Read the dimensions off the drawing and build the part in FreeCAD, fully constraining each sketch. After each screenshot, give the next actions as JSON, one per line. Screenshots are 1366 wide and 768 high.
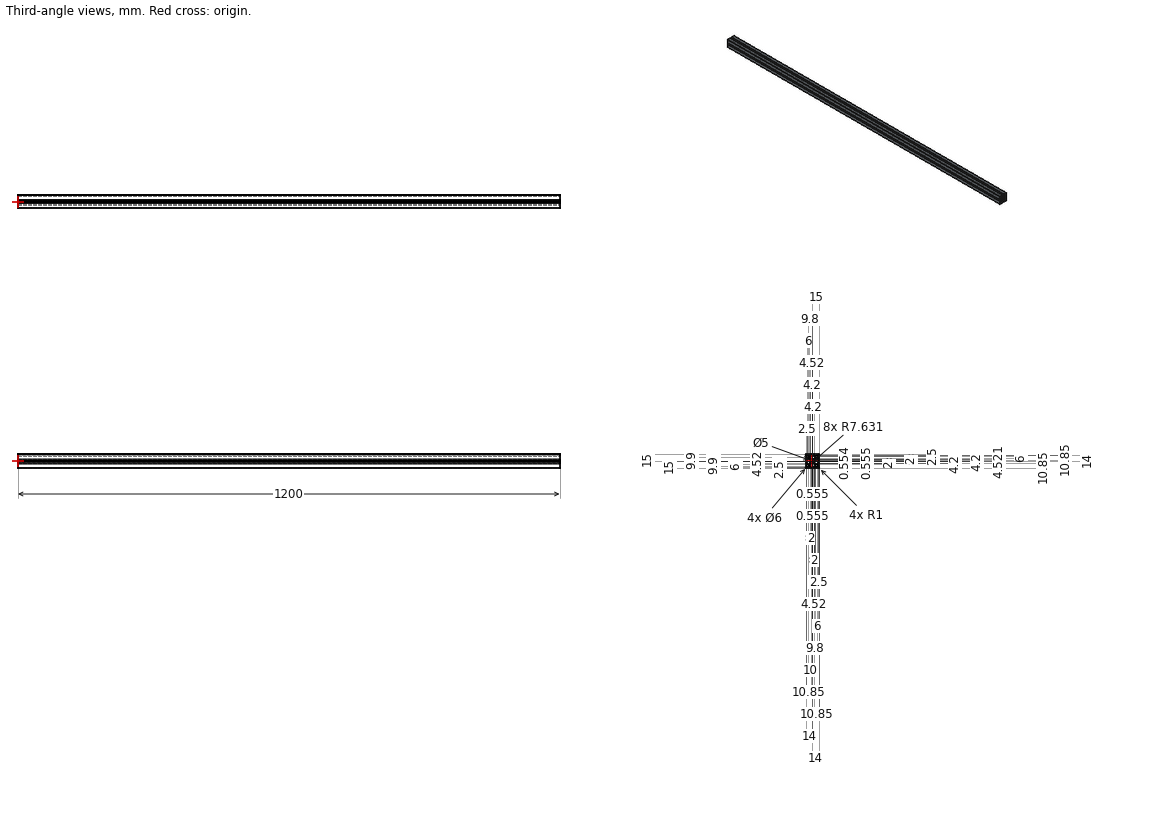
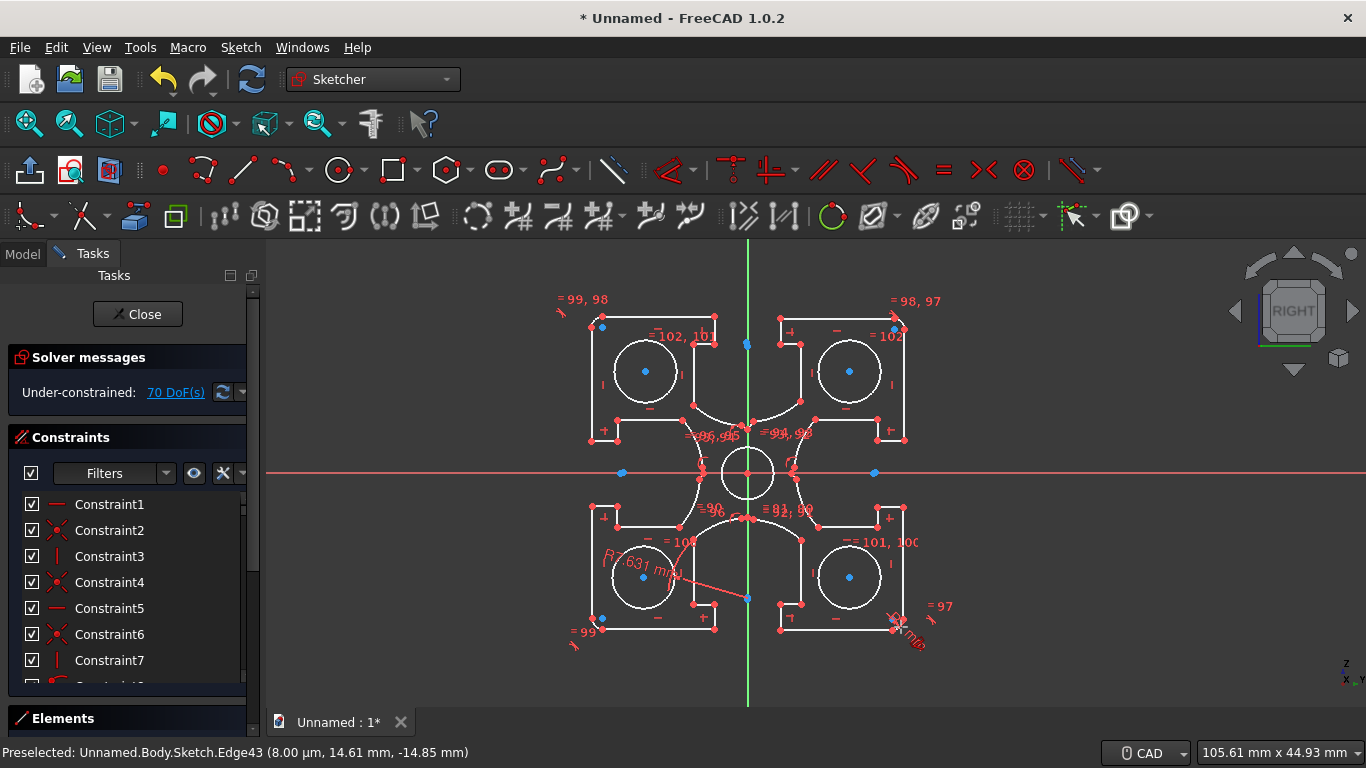
{"action": "left_click", "coordinate": [665, 555]}
{"action": "left_click", "coordinate": [726, 551]}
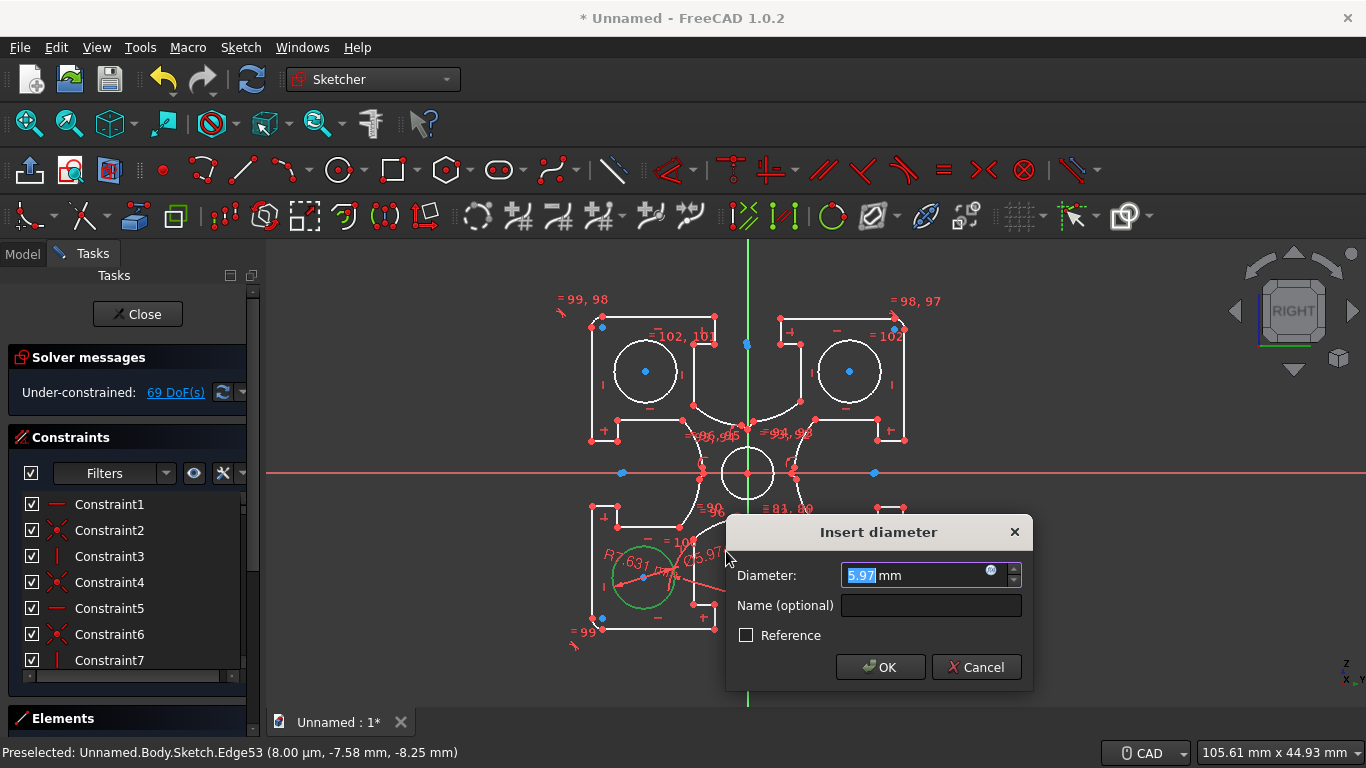
{"action": "type", "text": "6"}
{"action": "key", "text": "Return"}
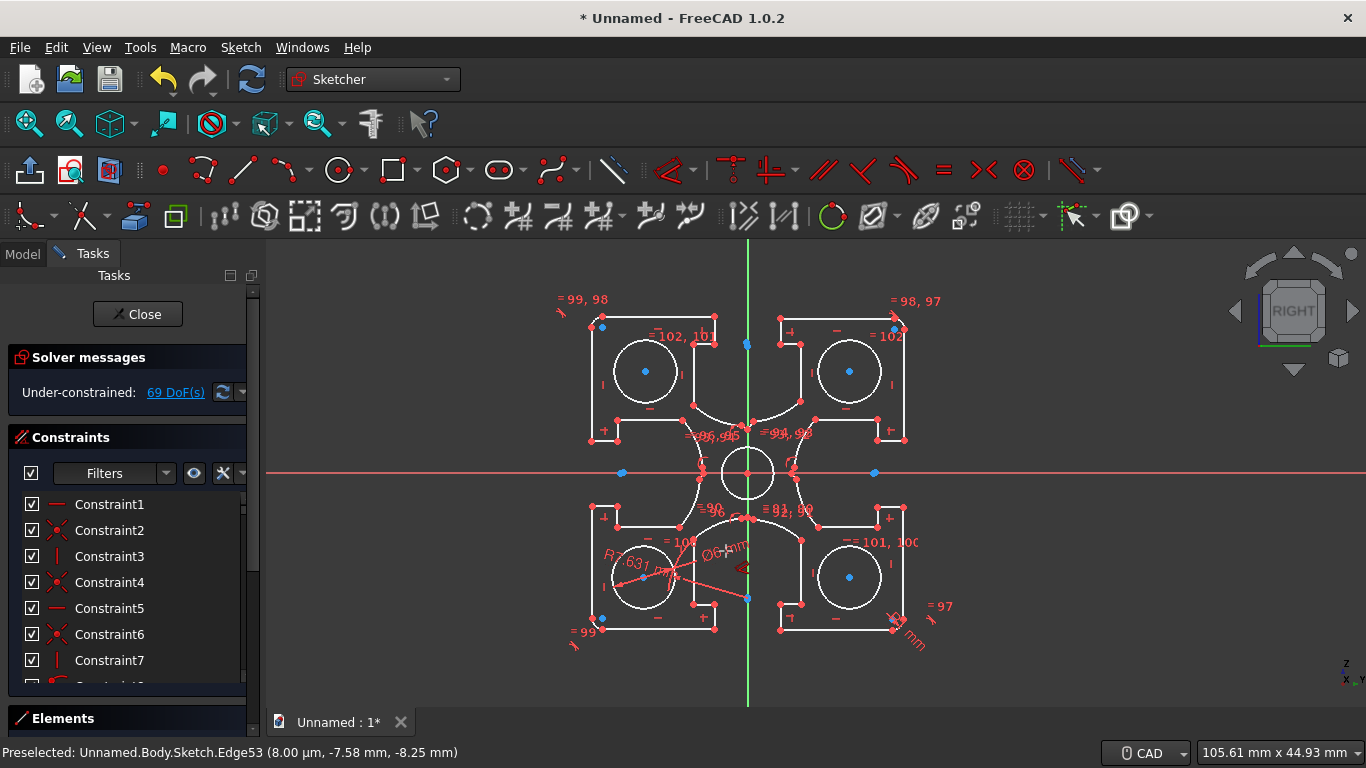
{"action": "left_click", "coordinate": [766, 455]}
{"action": "left_click", "coordinate": [789, 432]}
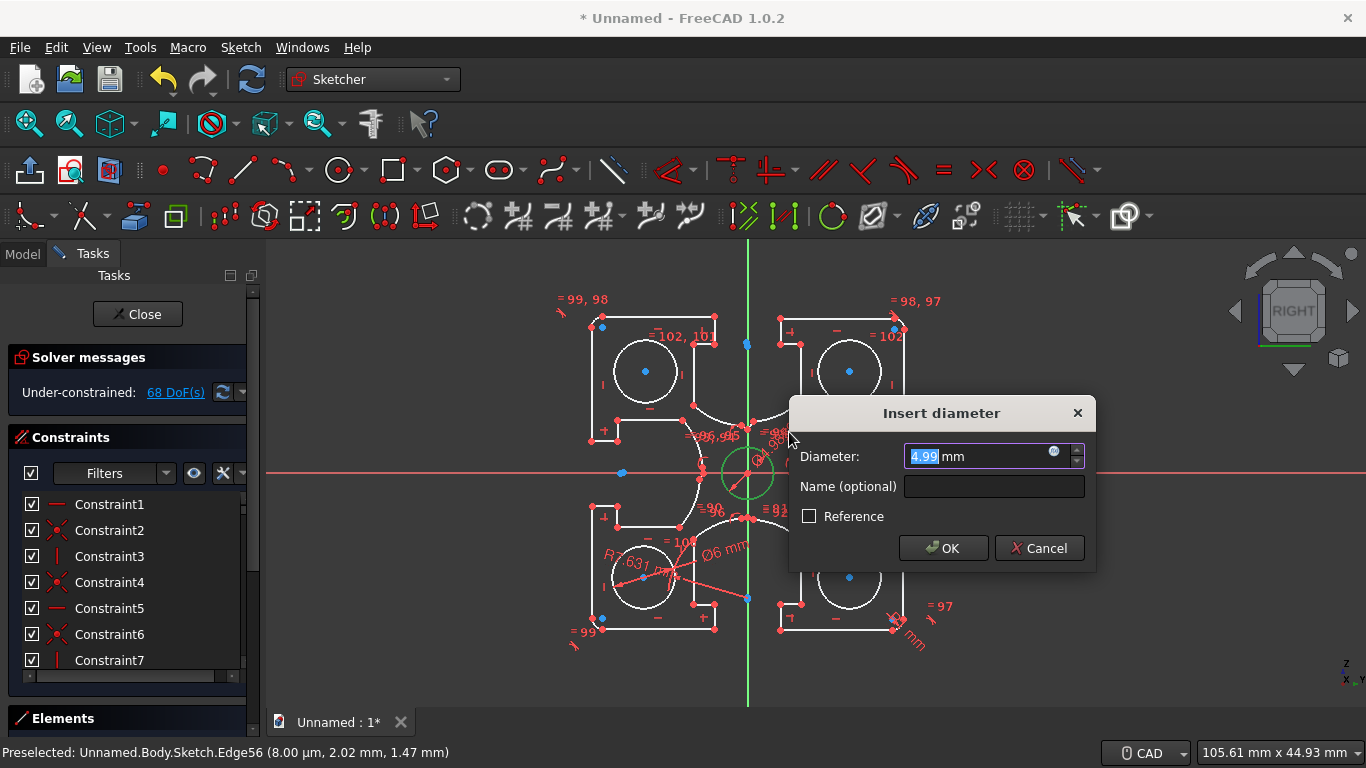
{"action": "type", "text": "5"}
{"action": "key", "text": "Return"}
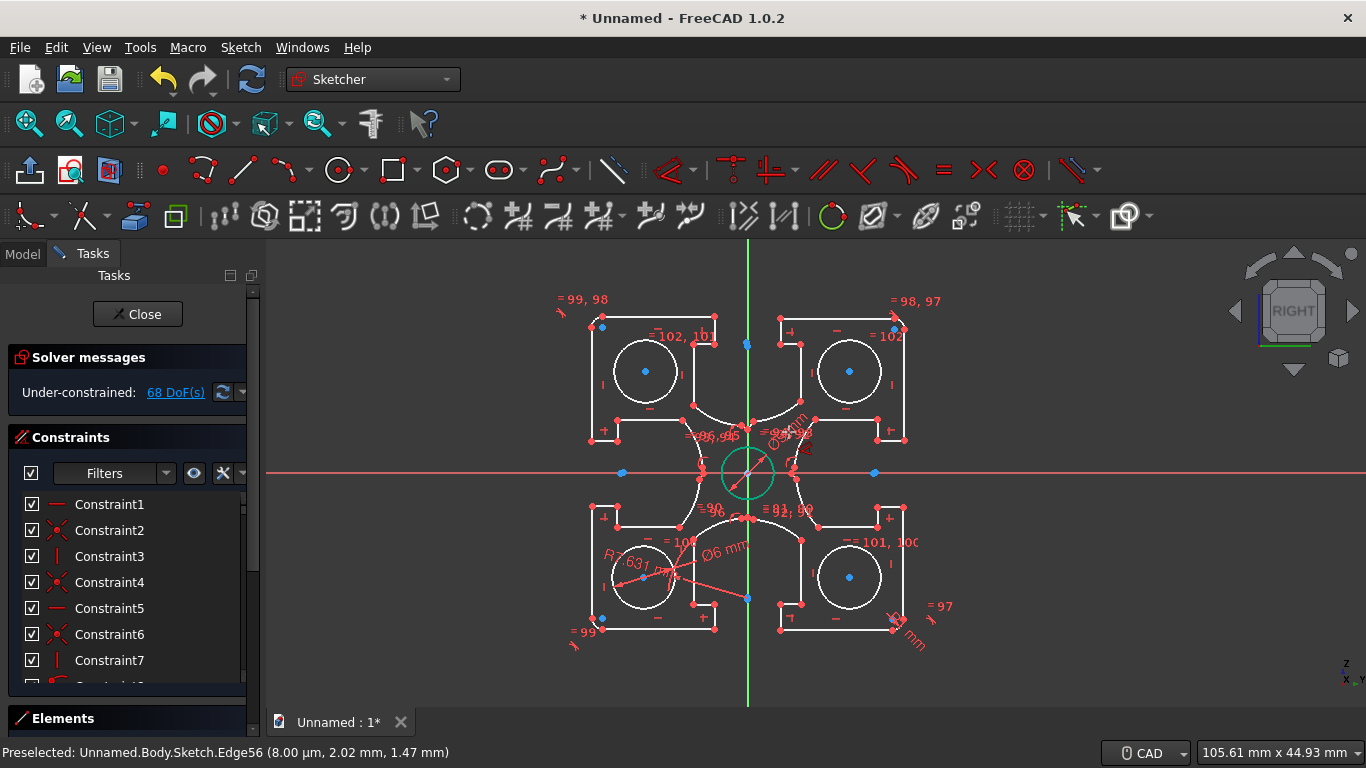
{"action": "scroll", "coordinate": [704, 605], "scroll_direction": "up", "scroll_amount": 4}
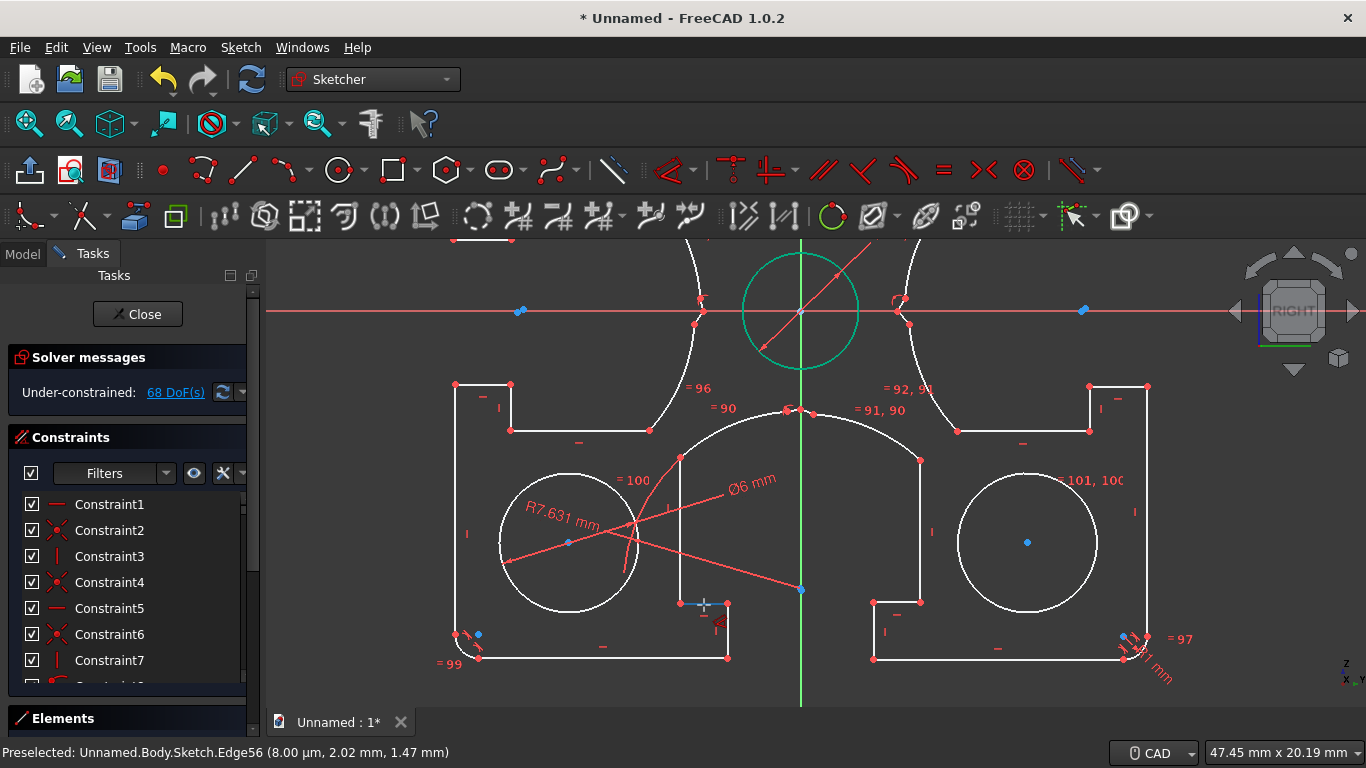
{"action": "left_click", "coordinate": [704, 604]}
{"action": "left_click", "coordinate": [704, 638]}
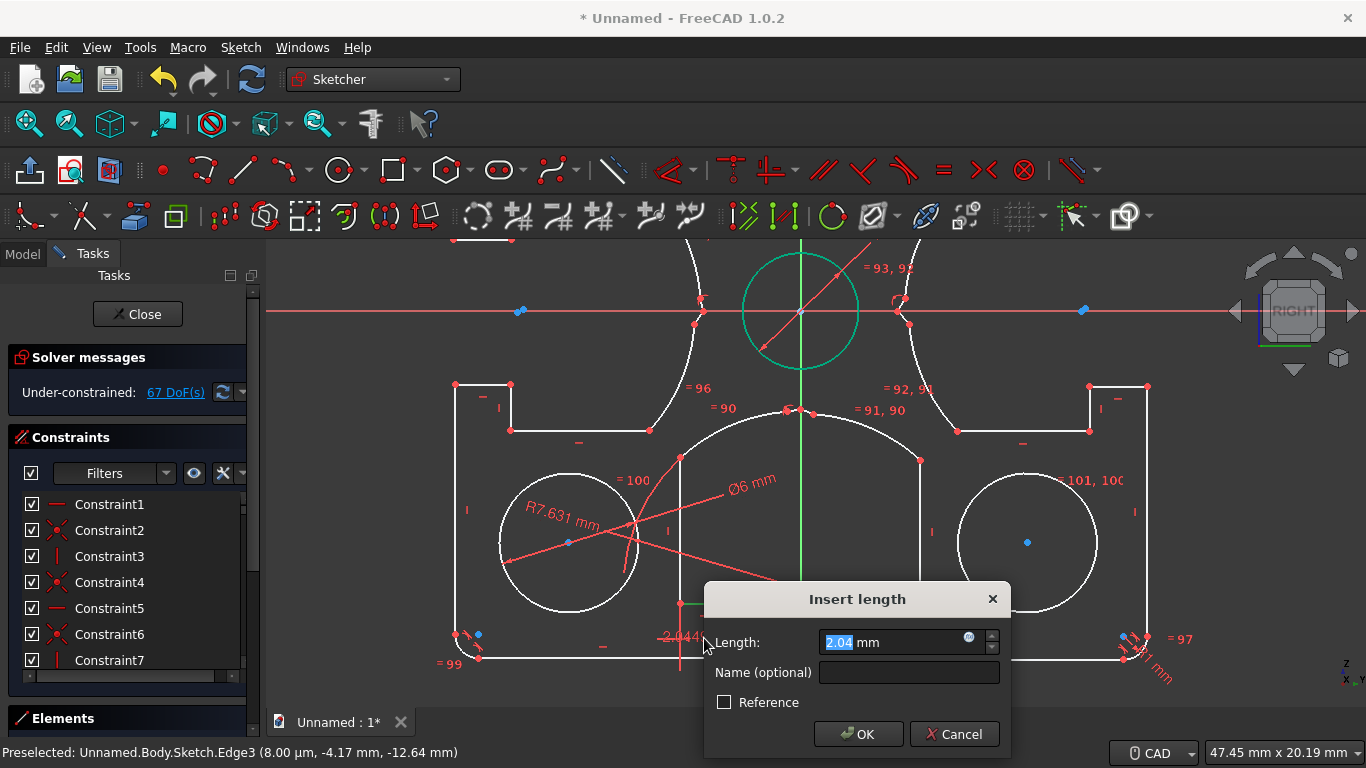
{"action": "type", "text": "2"}
{"action": "key", "text": "Return"}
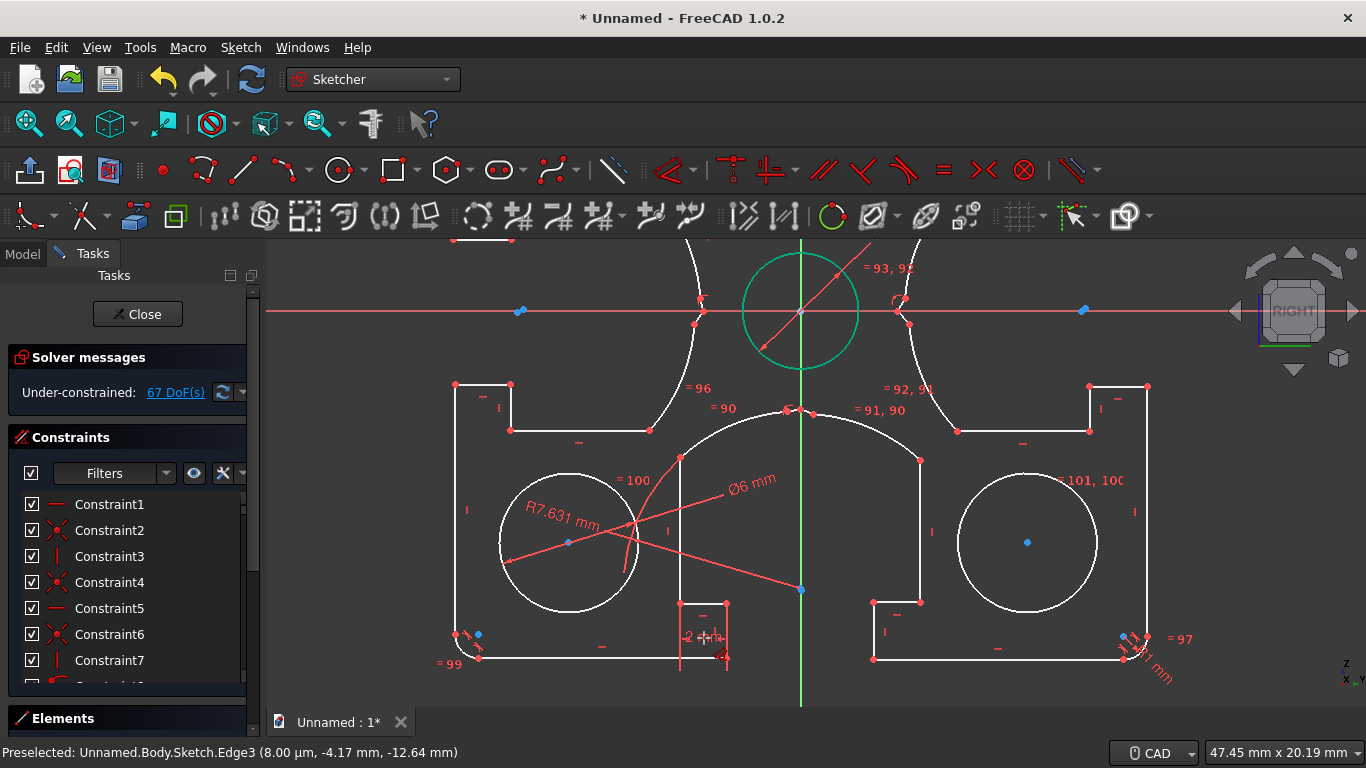
{"action": "left_click", "coordinate": [680, 560]}
{"action": "left_click", "coordinate": [646, 497]}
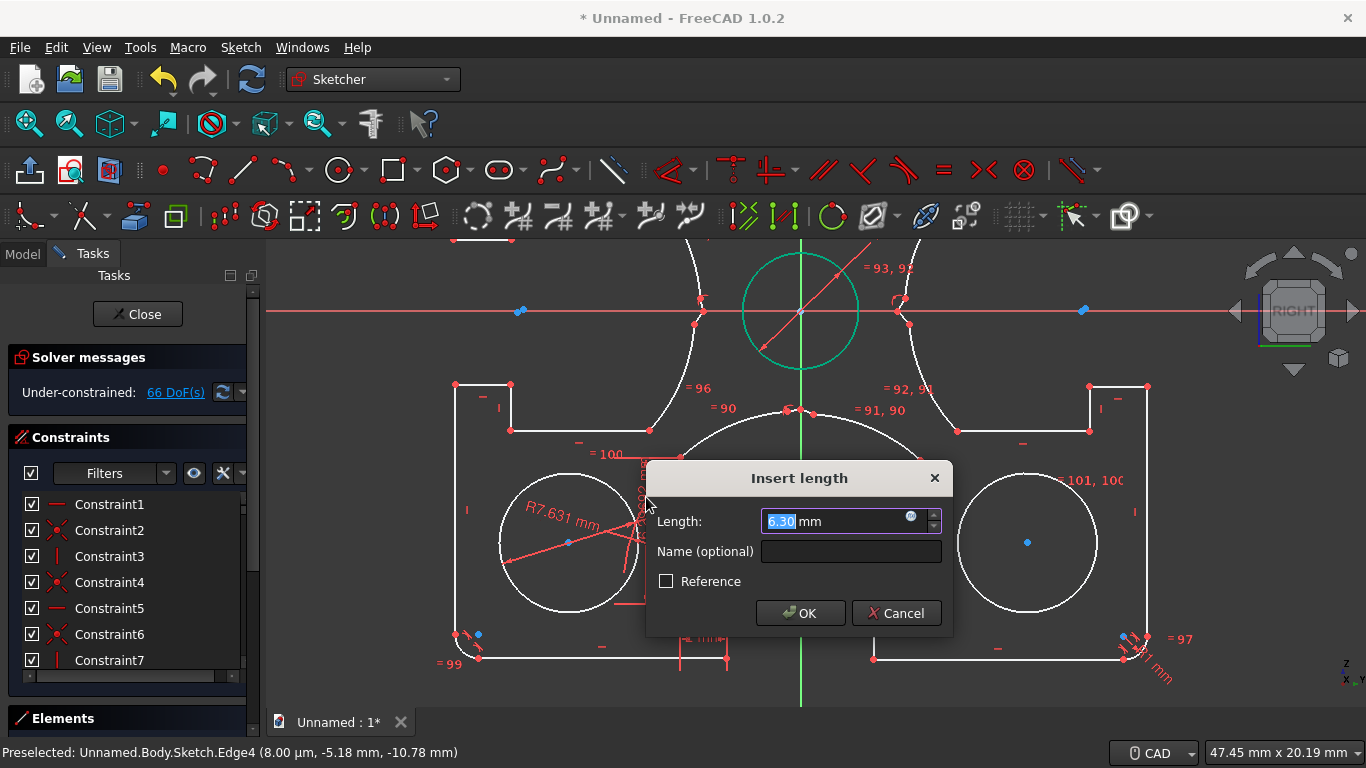
{"action": "type", "text": "6"}
{"action": "key", "text": "Return"}